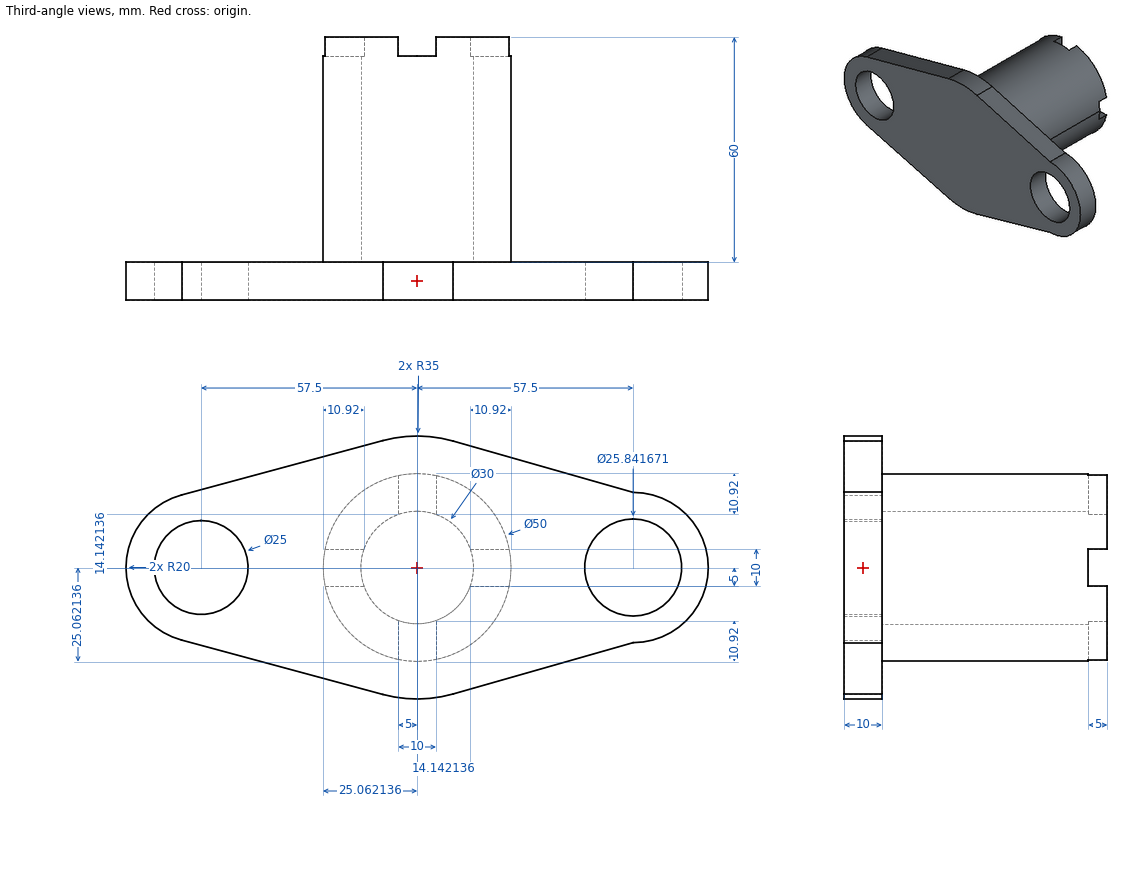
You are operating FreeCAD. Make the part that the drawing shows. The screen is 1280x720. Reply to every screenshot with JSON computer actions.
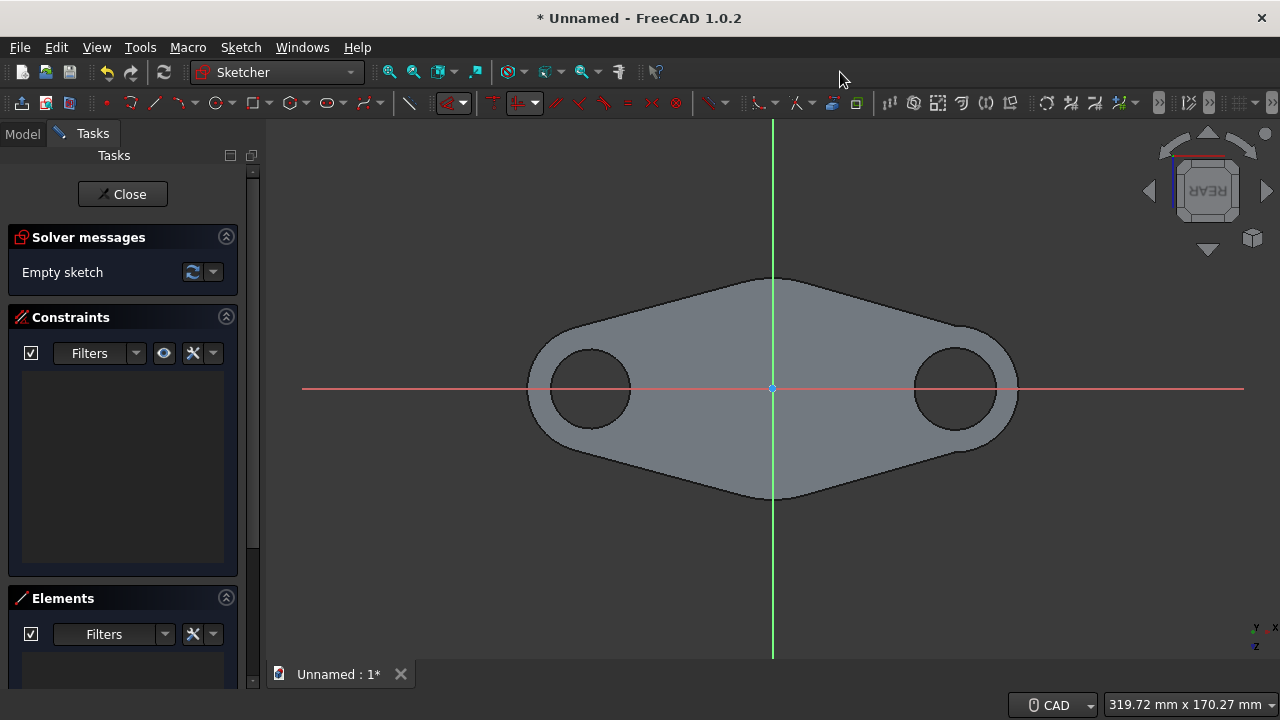
{"action": "scroll", "coordinate": [829, 389], "scroll_direction": "up", "scroll_amount": 4}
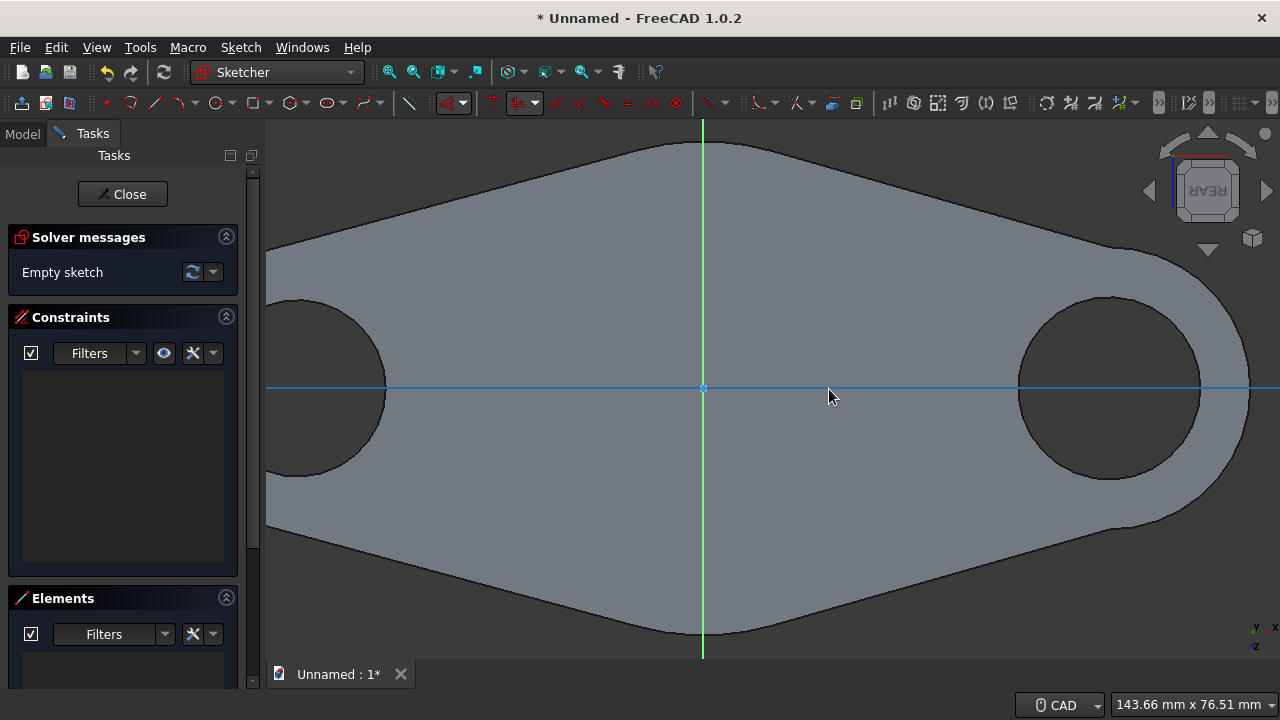
{"action": "key", "text": "g c"}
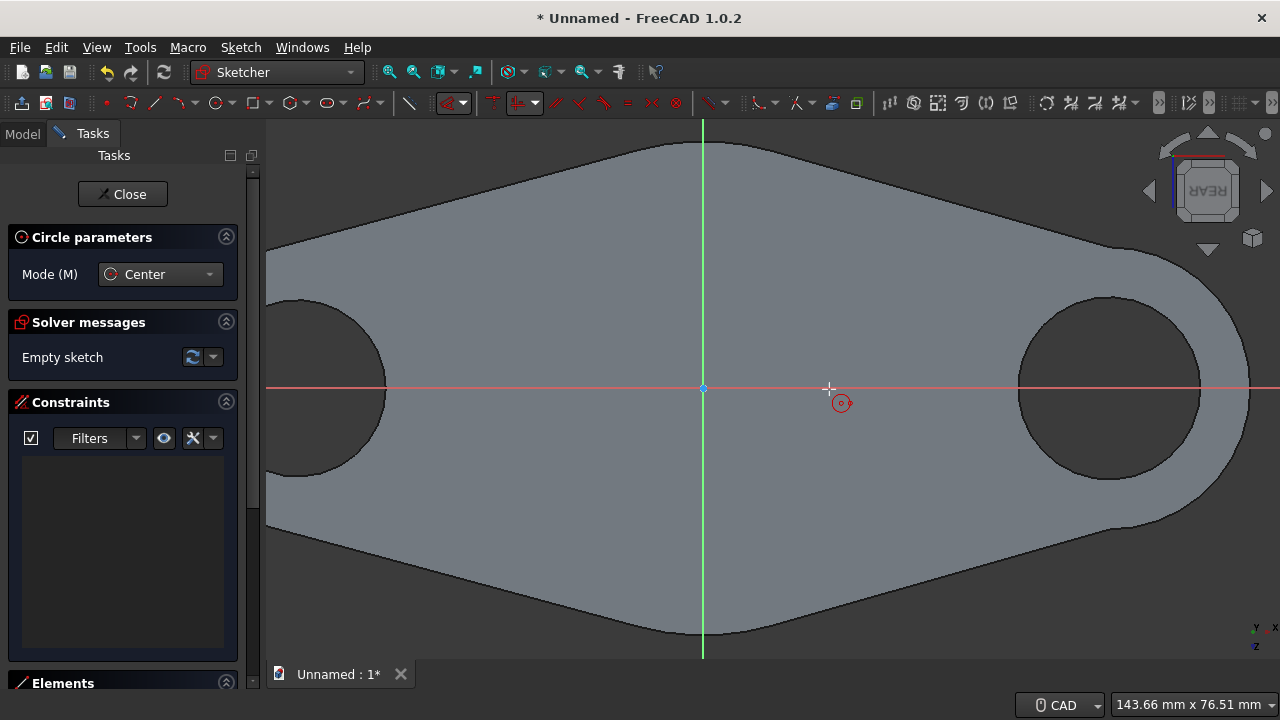
{"action": "left_click", "coordinate": [703, 388]}
{"action": "mouse_move", "coordinate": [828, 264]}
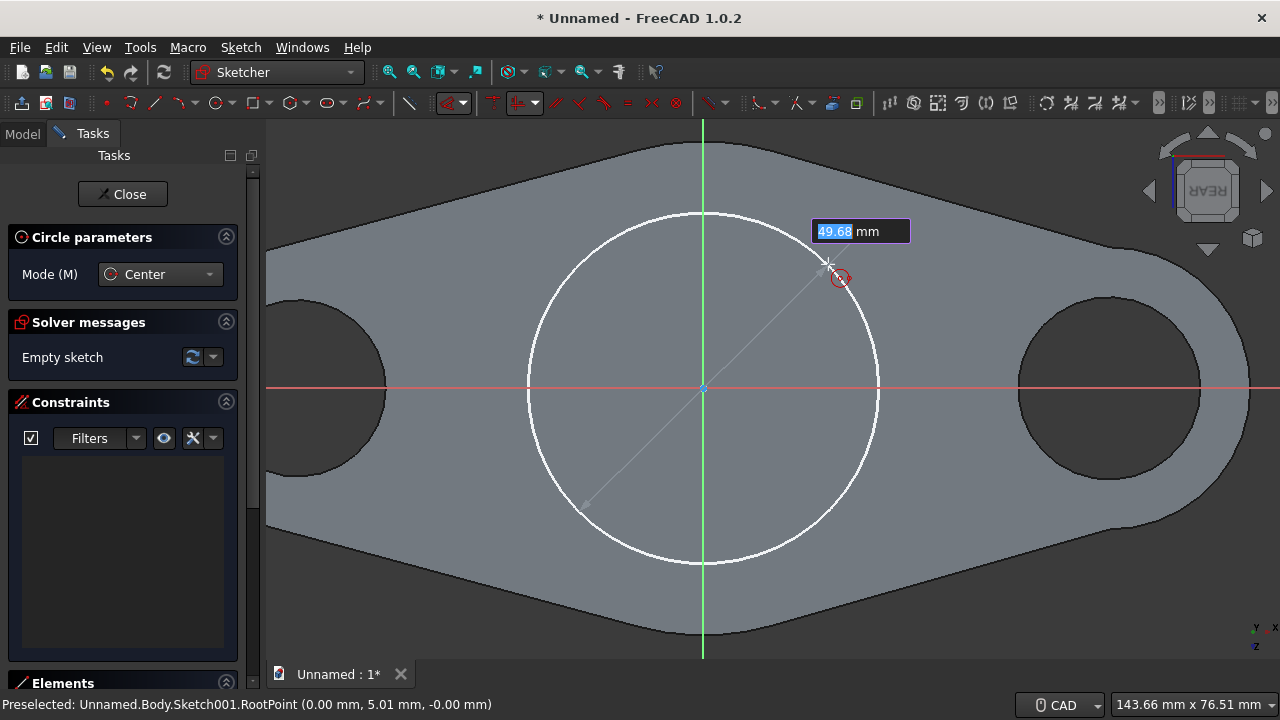
{"action": "type", "text": "50"}
{"action": "key", "text": "Return"}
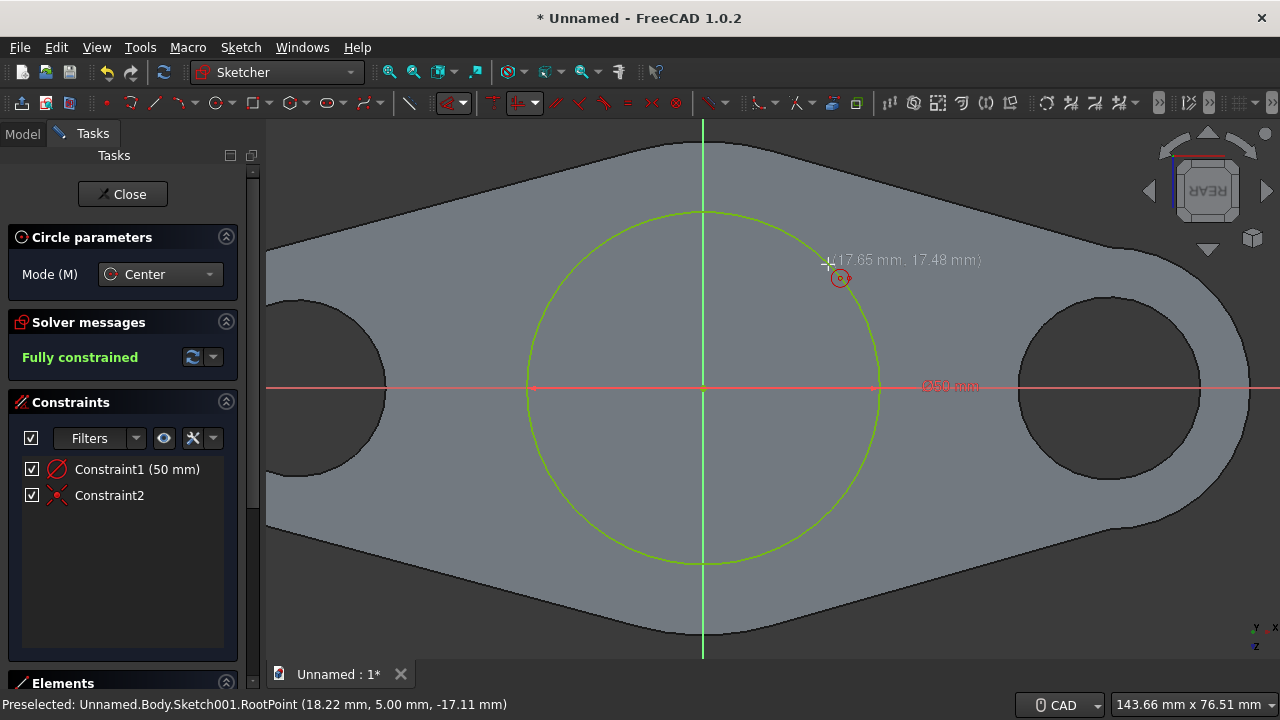
{"action": "left_click", "coordinate": [703, 388]}
{"action": "mouse_move", "coordinate": [778, 314]}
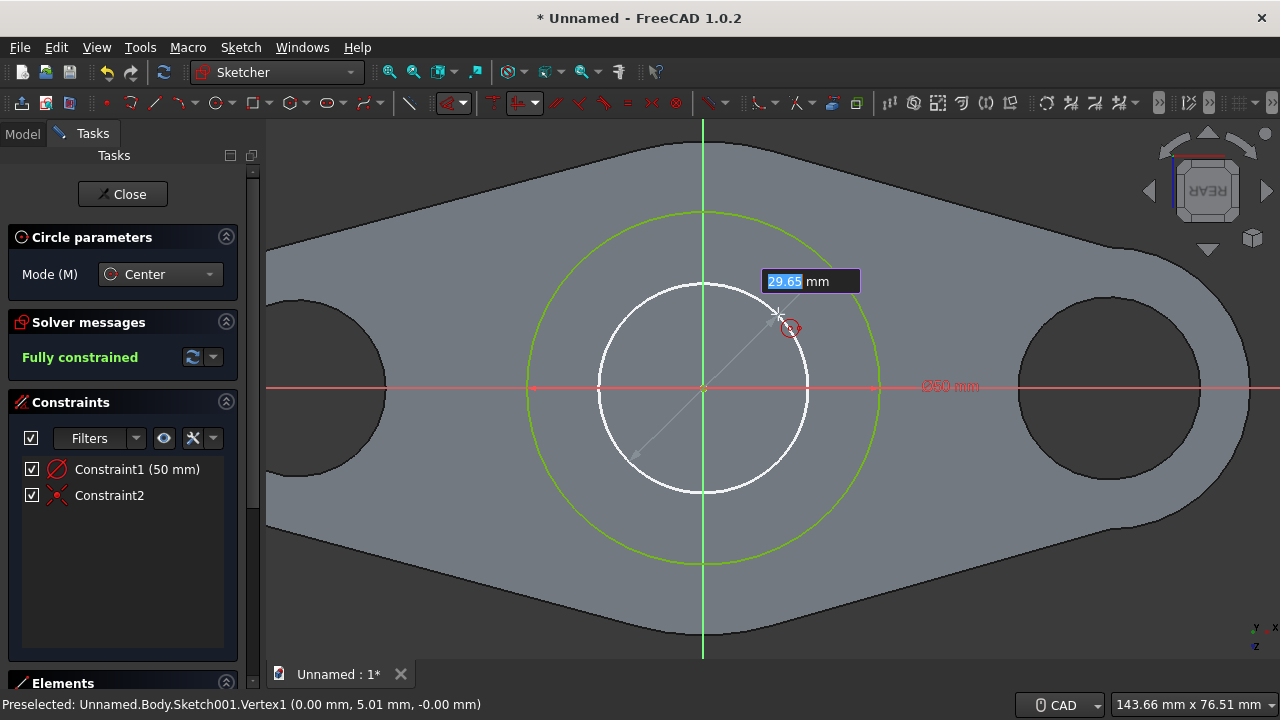
{"action": "type", "text": "30"}
{"action": "key", "text": "Return"}
{"action": "key", "text": "Escape"}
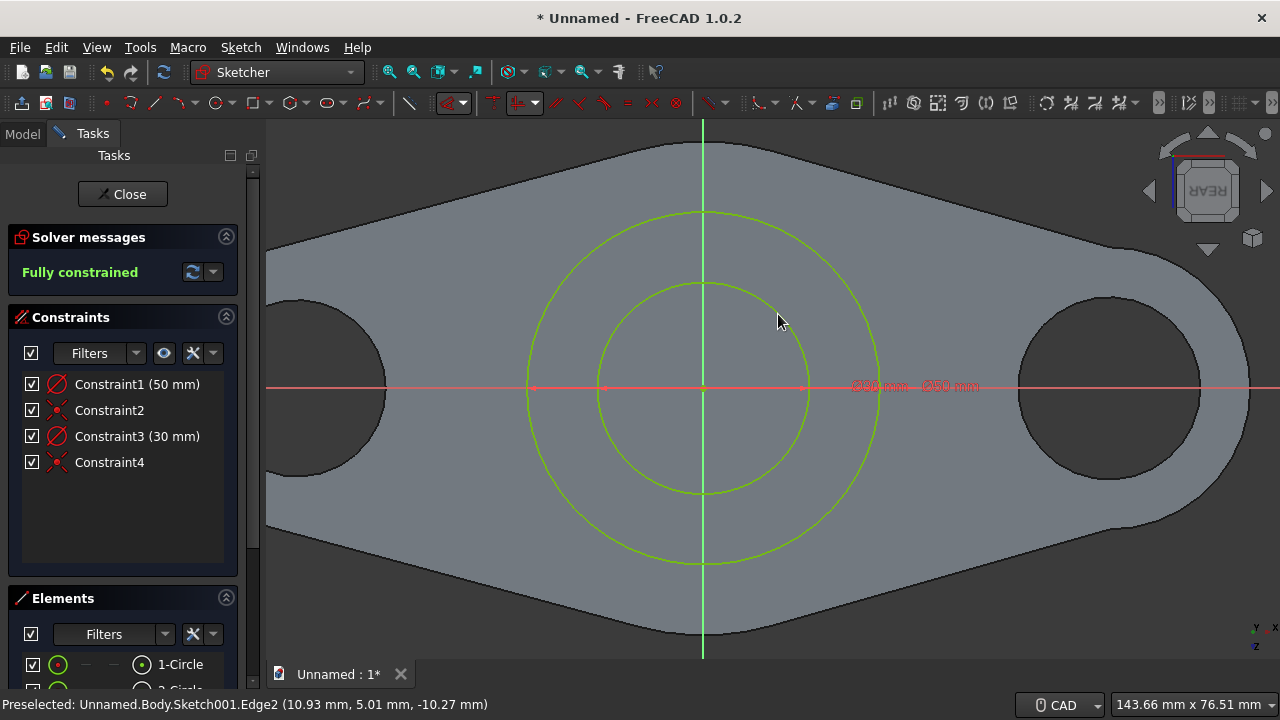
{"action": "left_click", "coordinate": [123, 194]}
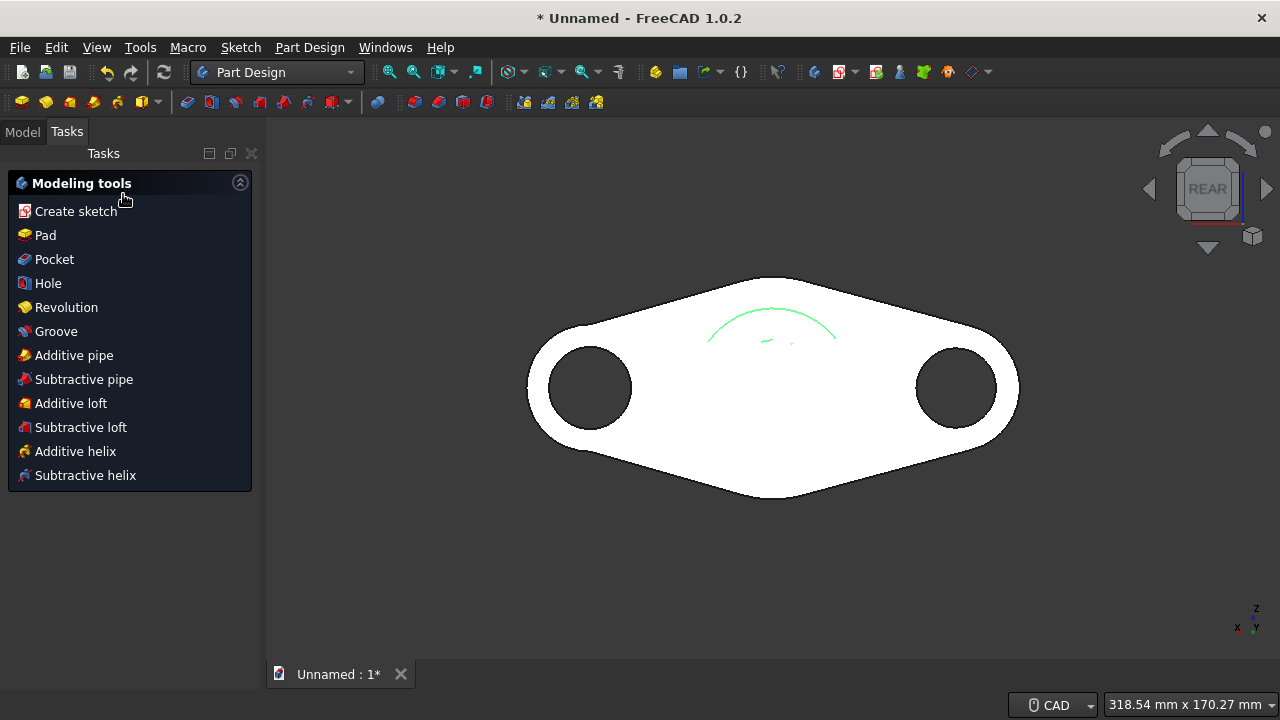
{"action": "left_click", "coordinate": [22, 102]}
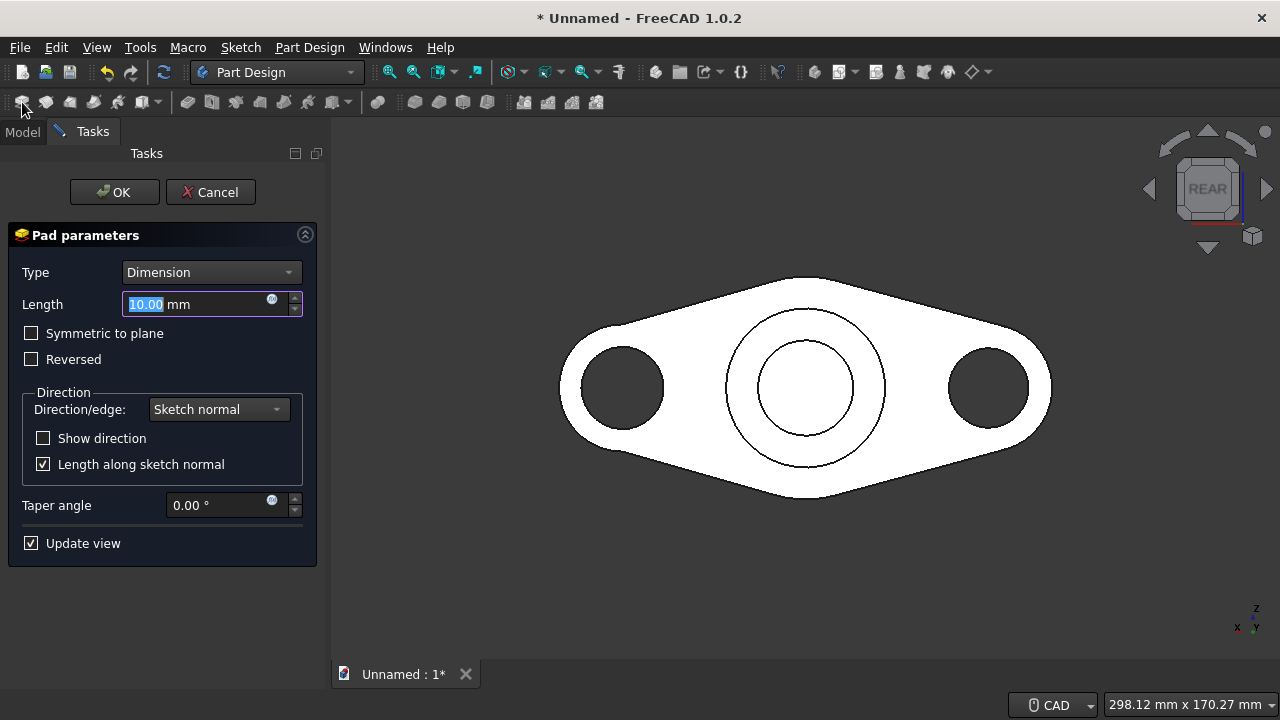
{"action": "type", "text": "60"}
{"action": "key", "text": "Tab"}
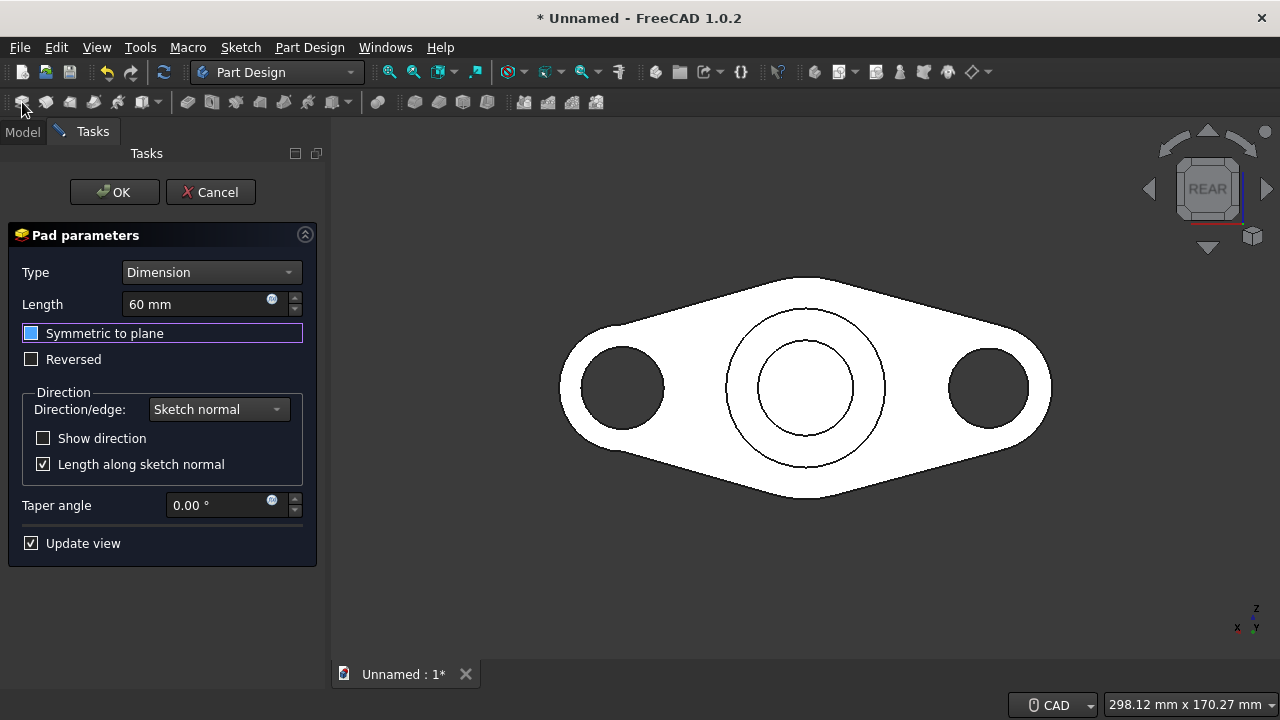
{"action": "left_click", "coordinate": [115, 192]}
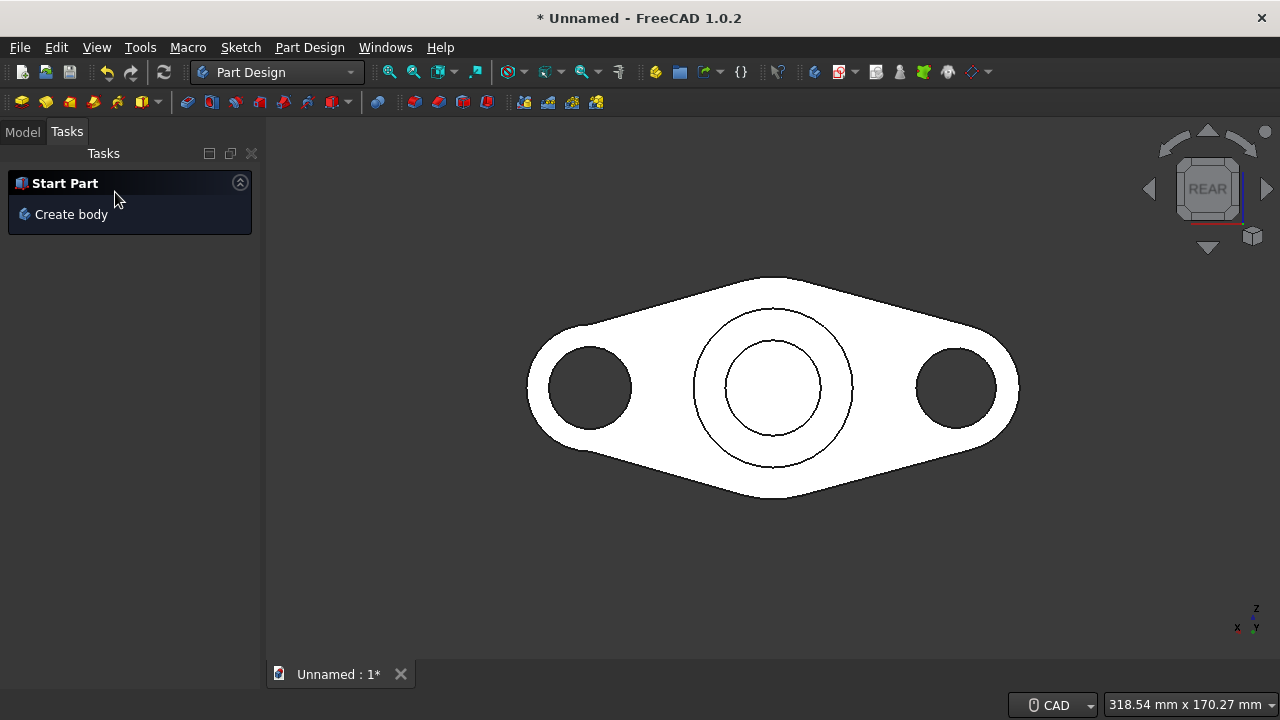
{"action": "left_click", "coordinate": [728, 342]}